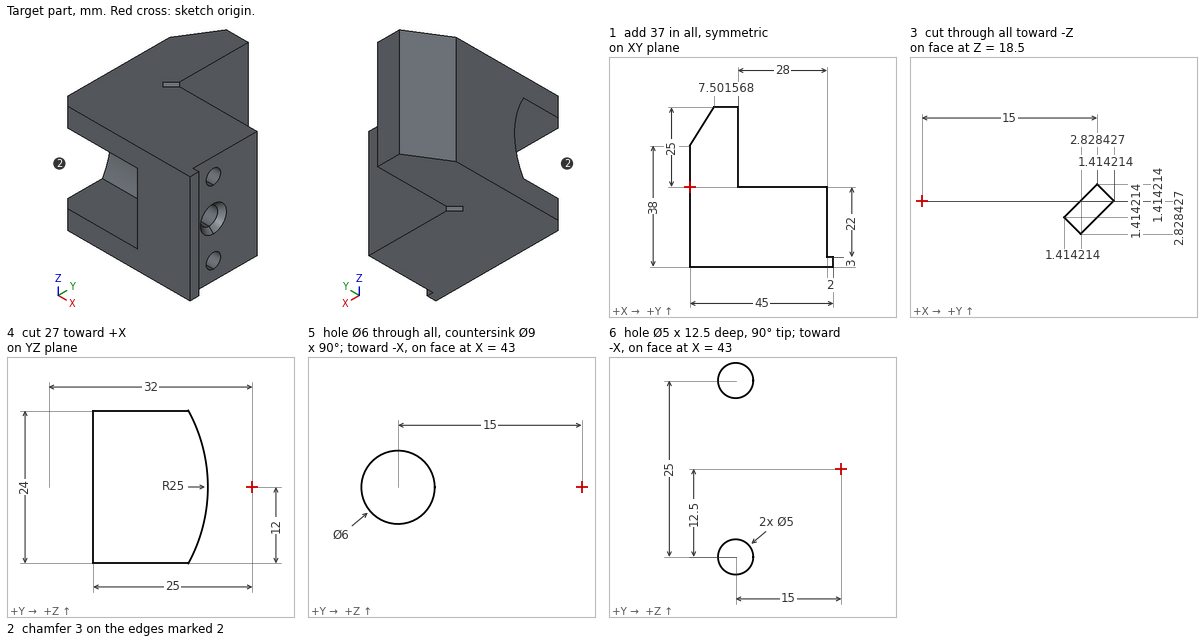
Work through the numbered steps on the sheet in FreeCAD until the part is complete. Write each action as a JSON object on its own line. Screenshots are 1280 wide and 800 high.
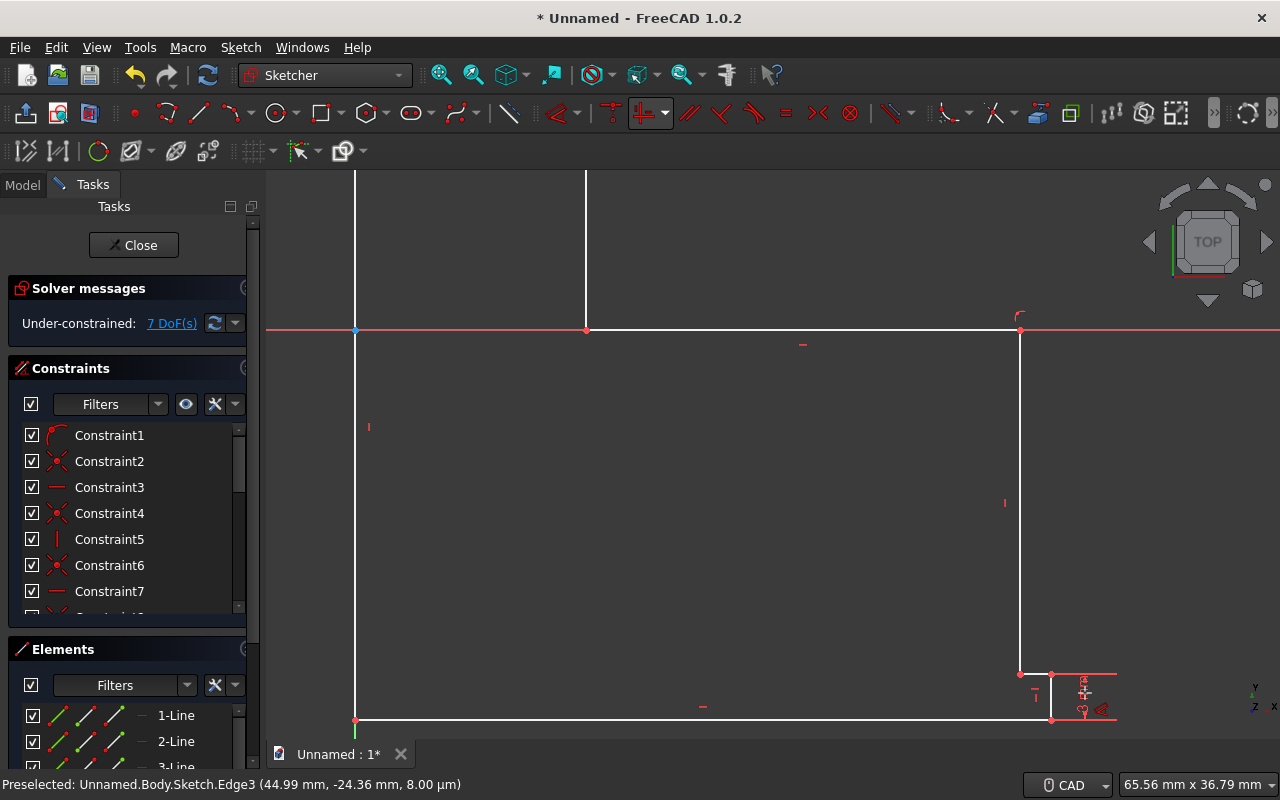
{"action": "scroll", "coordinate": [1042, 674], "scroll_direction": "up", "scroll_amount": 2}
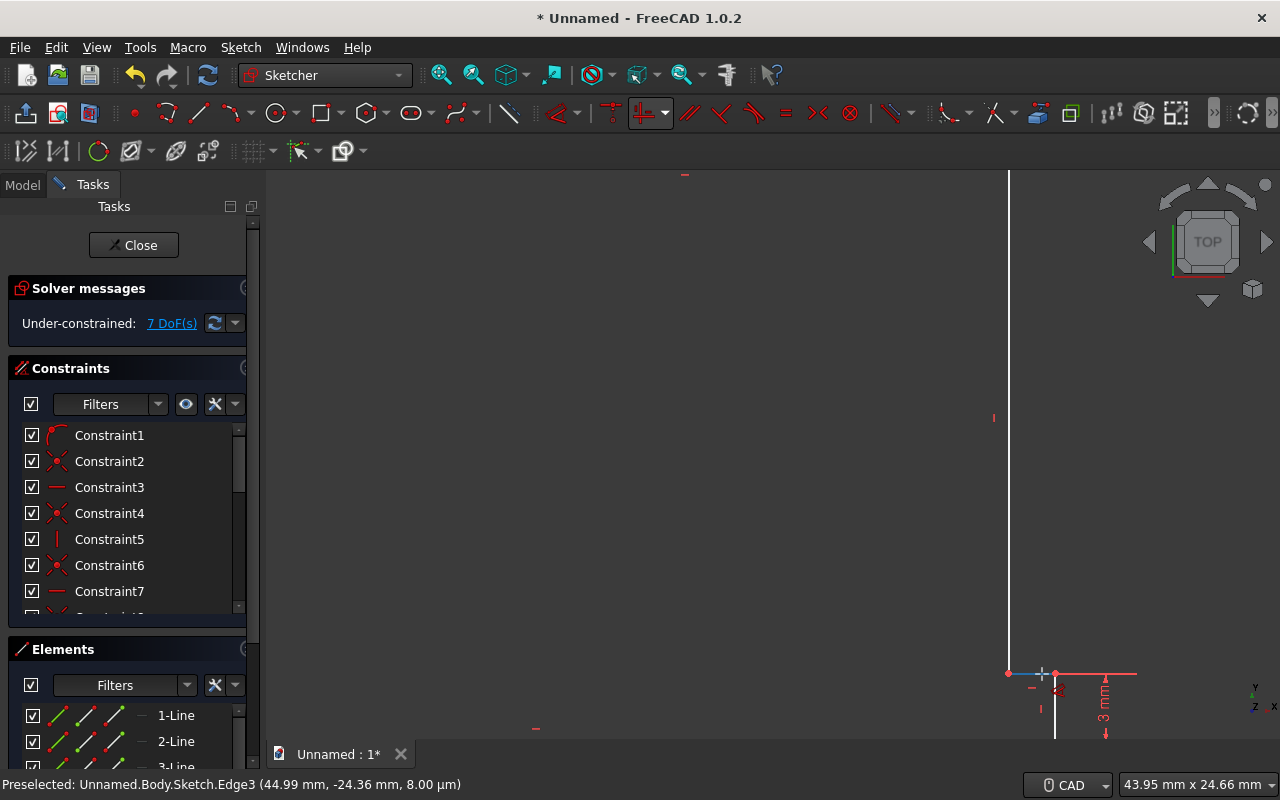
{"action": "left_click", "coordinate": [1041, 674]}
{"action": "left_click", "coordinate": [1032, 708]}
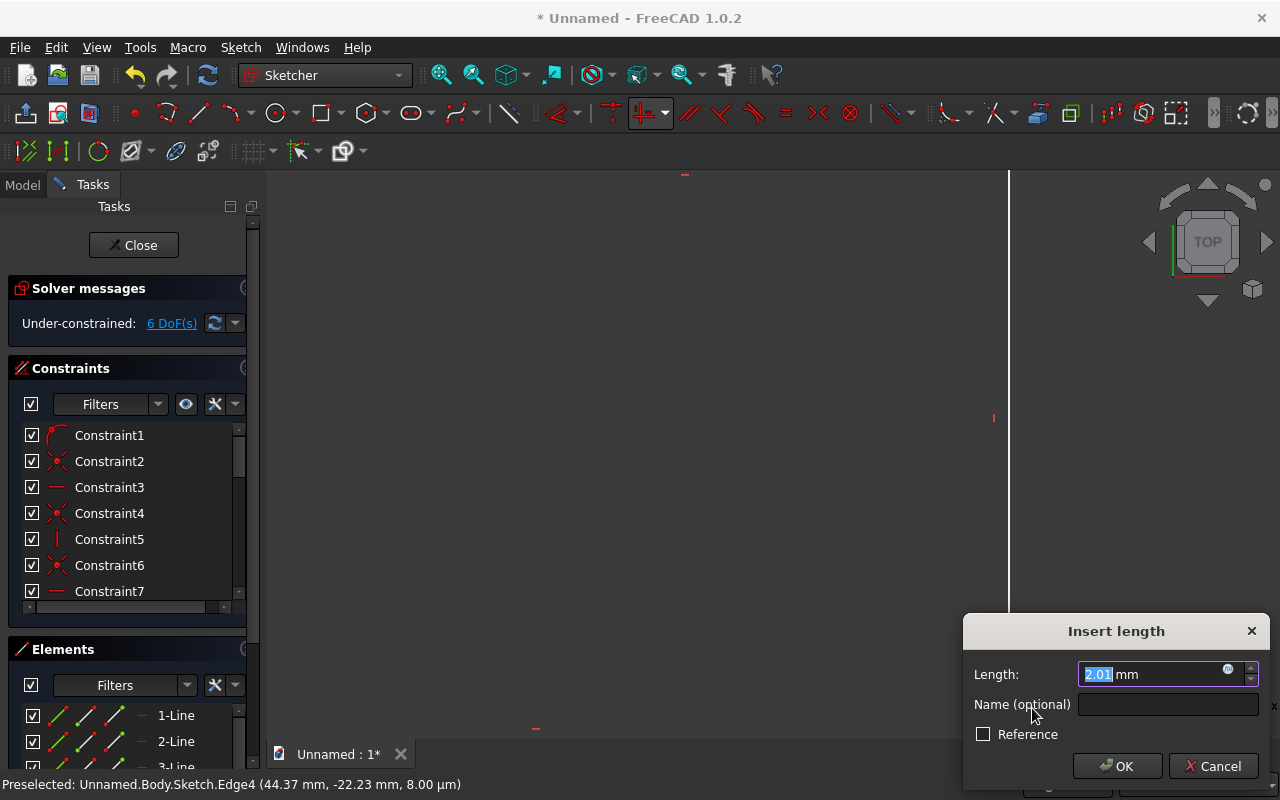
{"action": "type", "text": "2"}
{"action": "key", "text": "Return"}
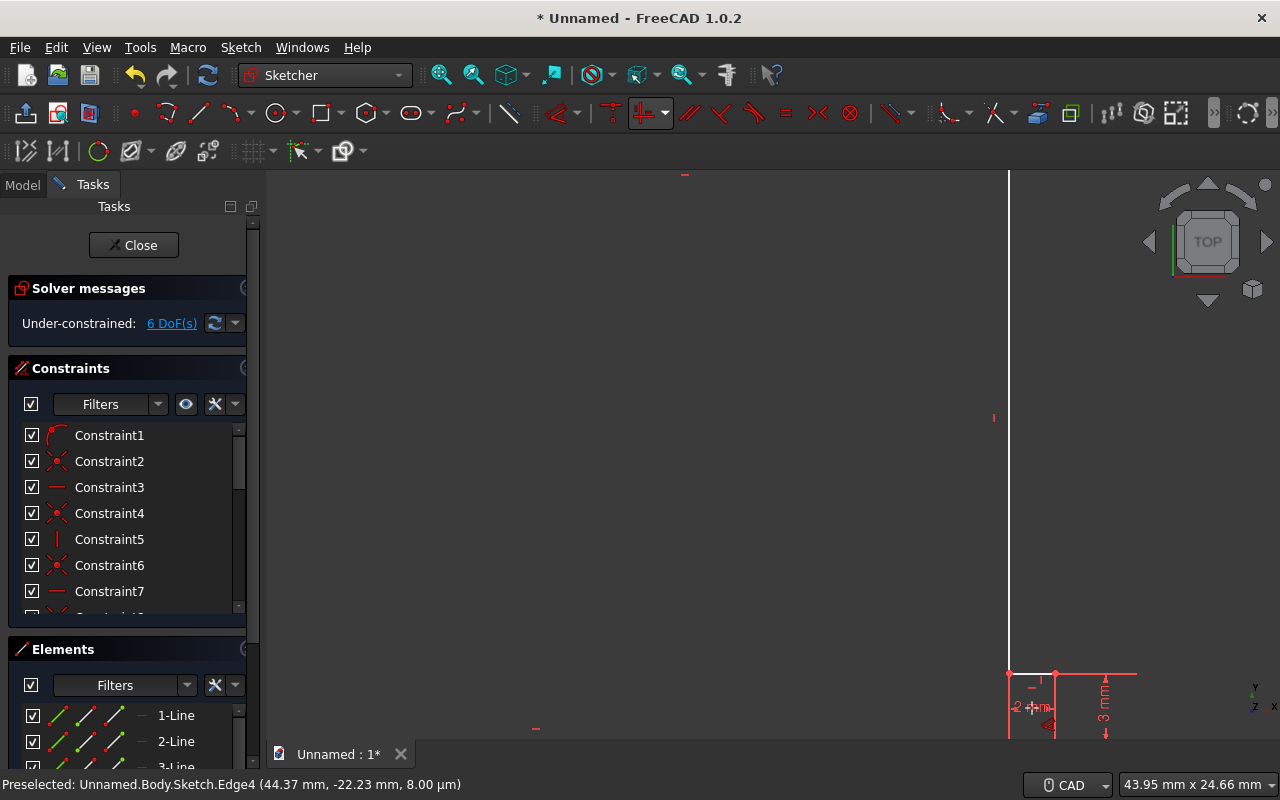
{"action": "scroll", "coordinate": [777, 581], "scroll_direction": "down", "scroll_amount": 6}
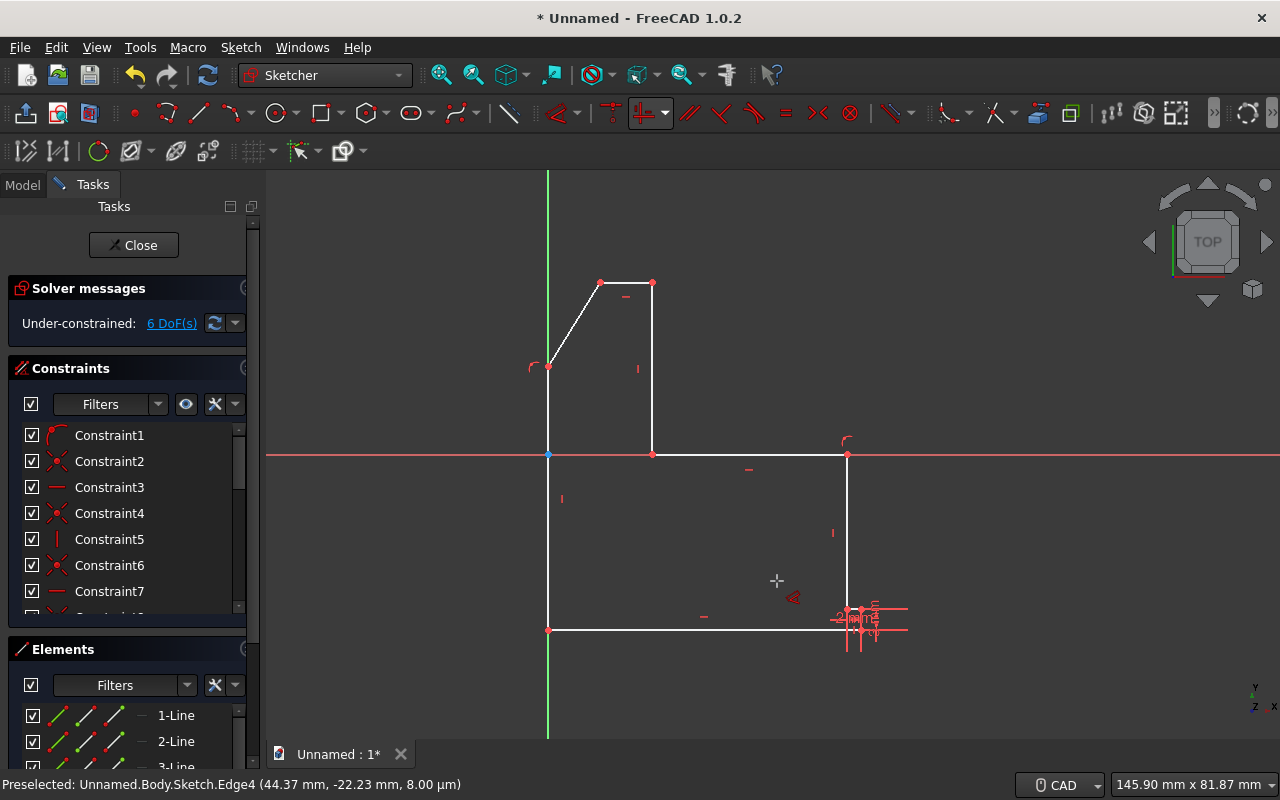
{"action": "scroll", "coordinate": [548, 446], "scroll_direction": "up", "scroll_amount": 2}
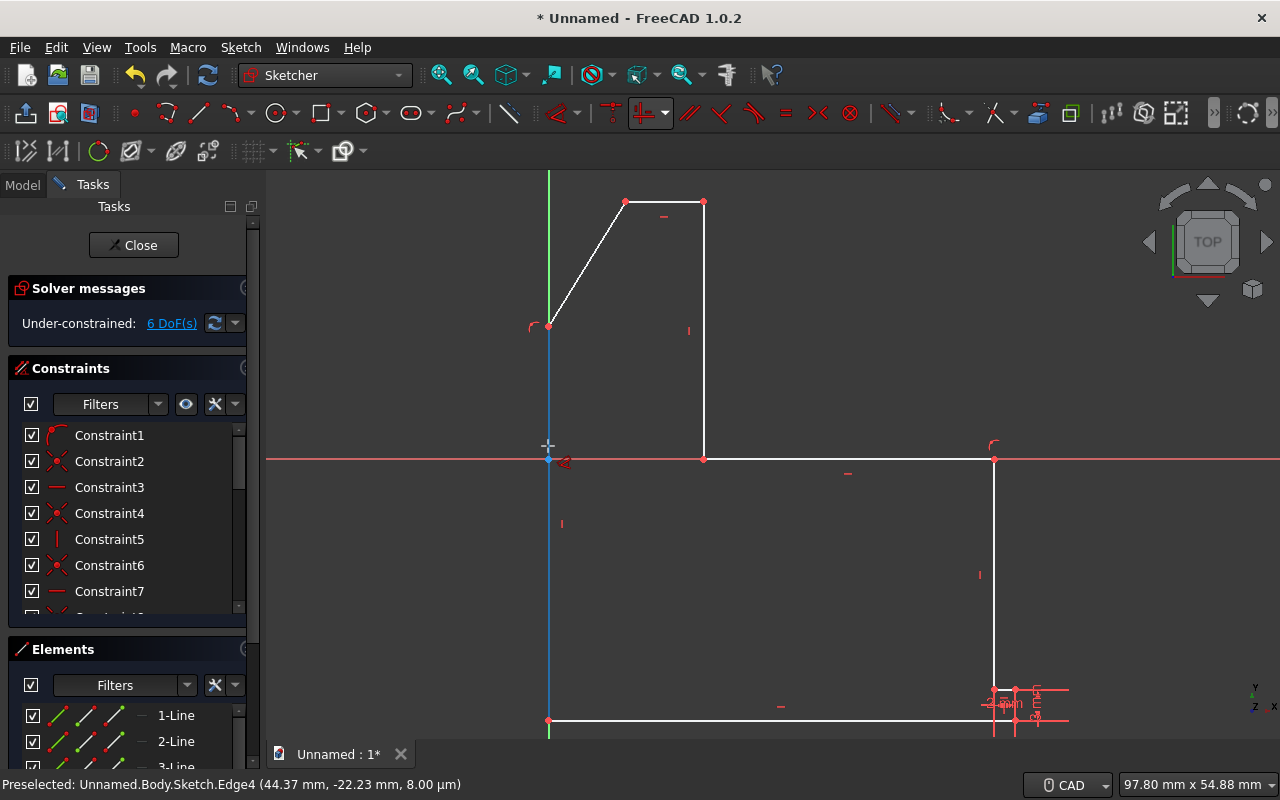
{"action": "left_click", "coordinate": [549, 445]}
{"action": "left_click", "coordinate": [515, 519]}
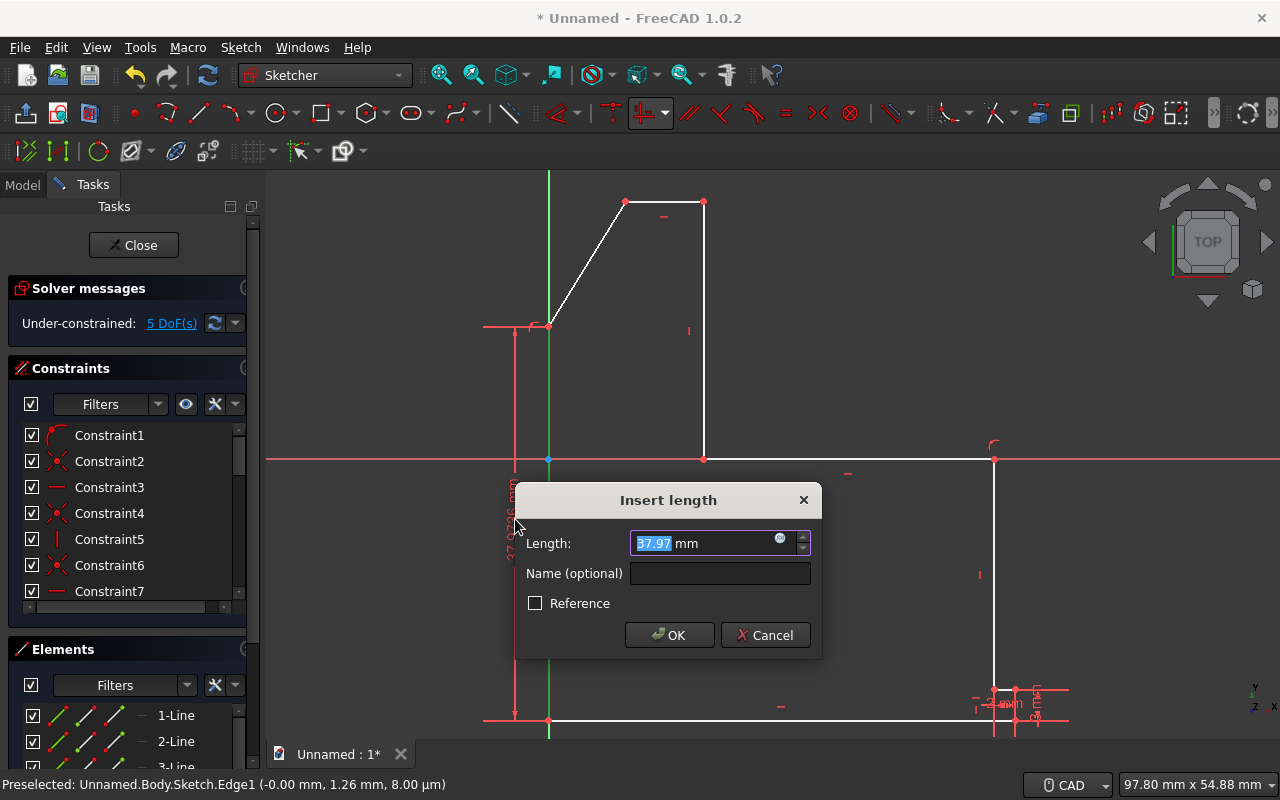
{"action": "type", "text": "38"}
{"action": "key", "text": "Return"}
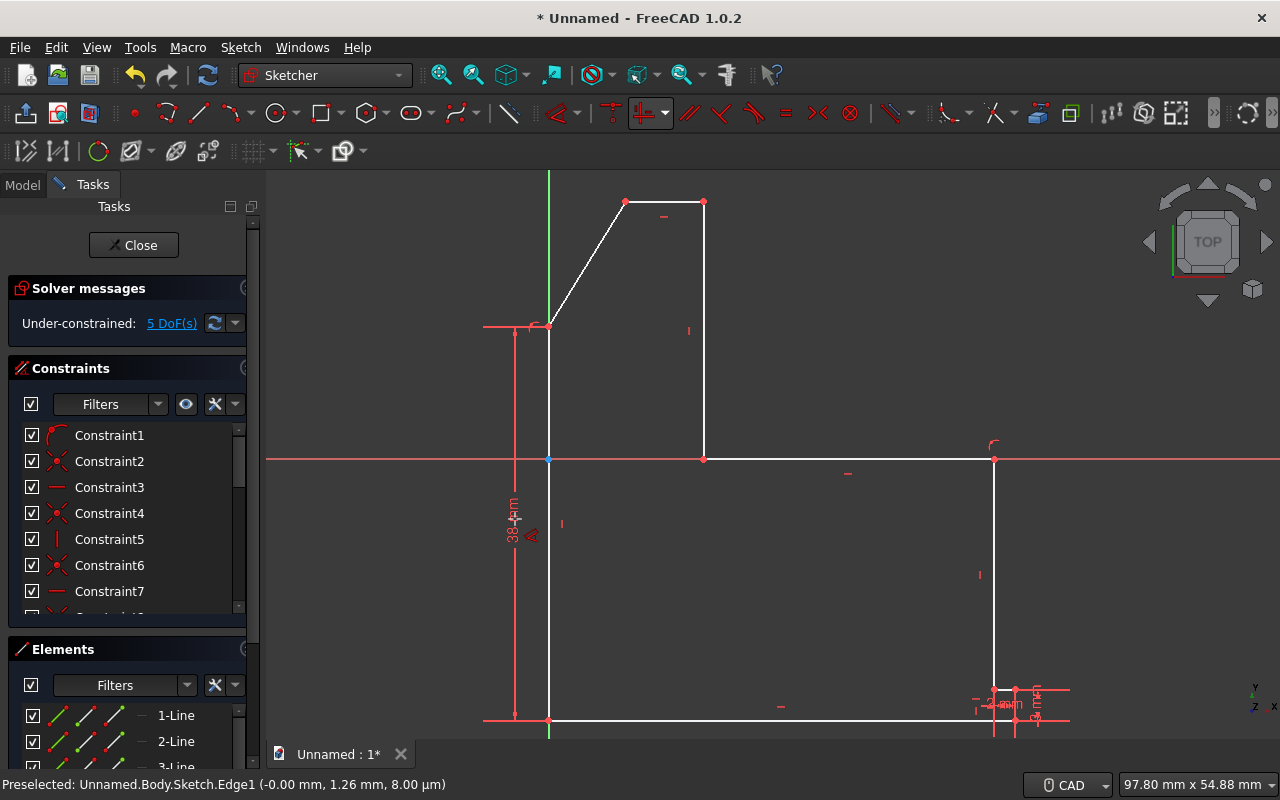
{"action": "scroll", "coordinate": [547, 445], "scroll_direction": "down", "scroll_amount": 2}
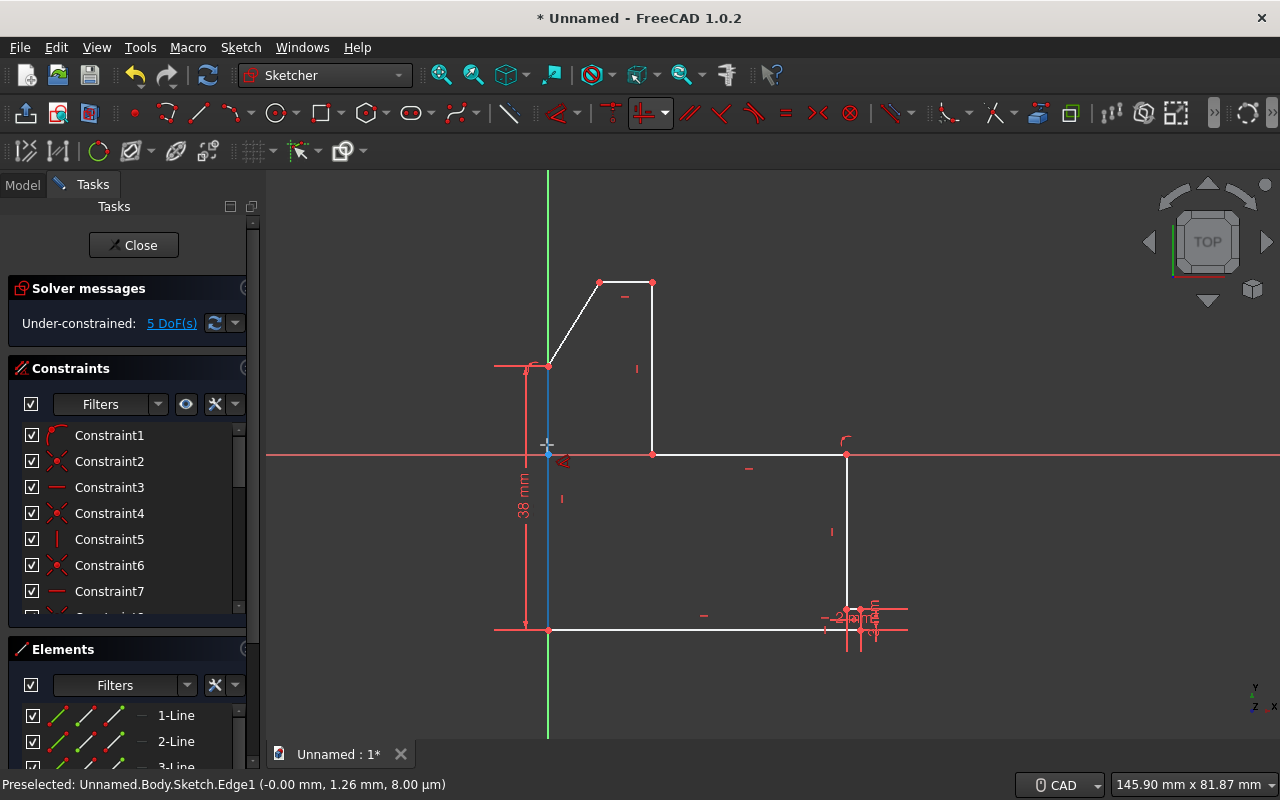
{"action": "left_click", "coordinate": [642, 630]}
{"action": "left_click", "coordinate": [704, 664]}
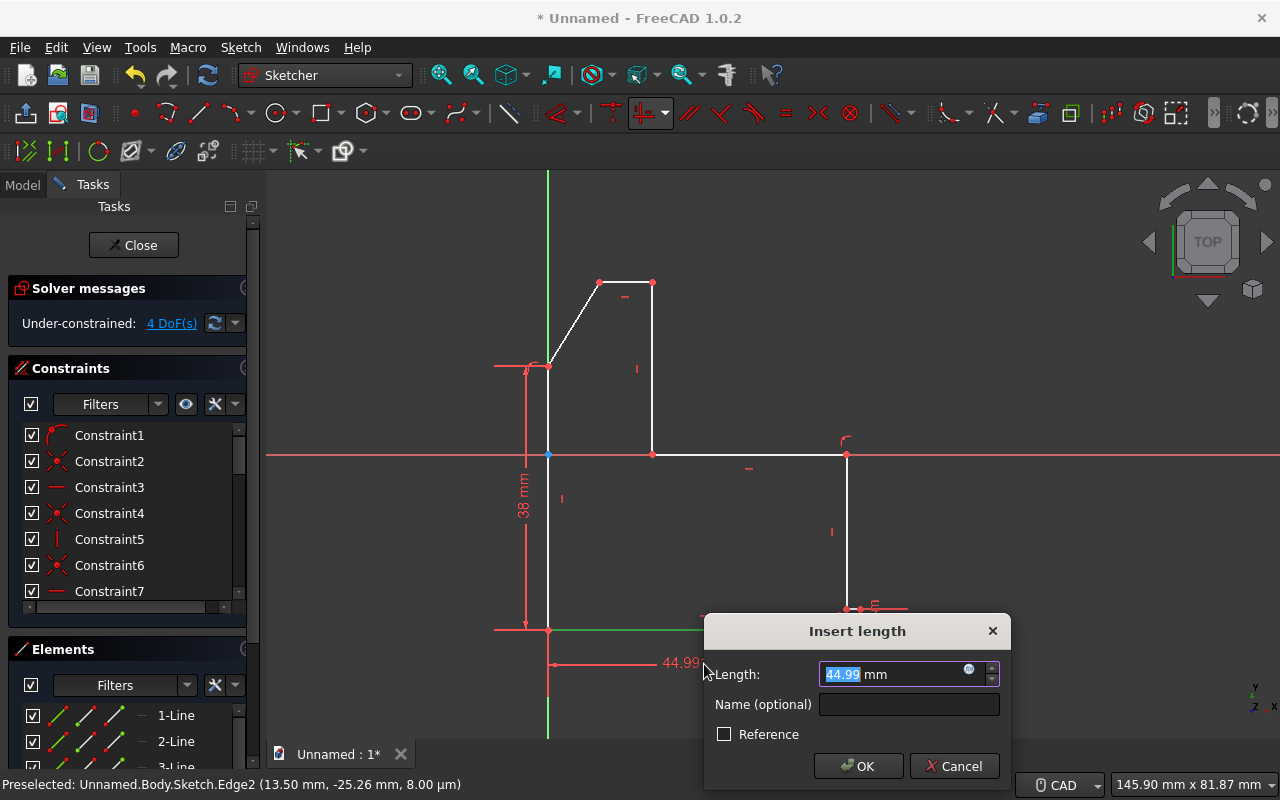
{"action": "type", "text": "45"}
{"action": "key", "text": "Return"}